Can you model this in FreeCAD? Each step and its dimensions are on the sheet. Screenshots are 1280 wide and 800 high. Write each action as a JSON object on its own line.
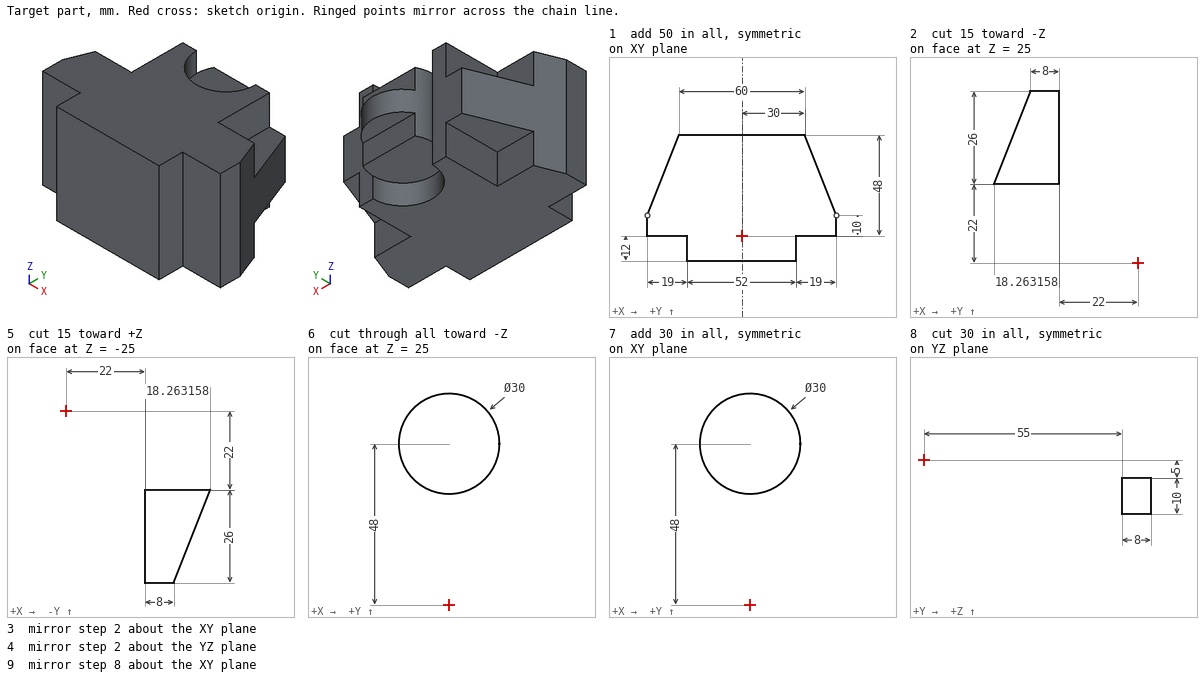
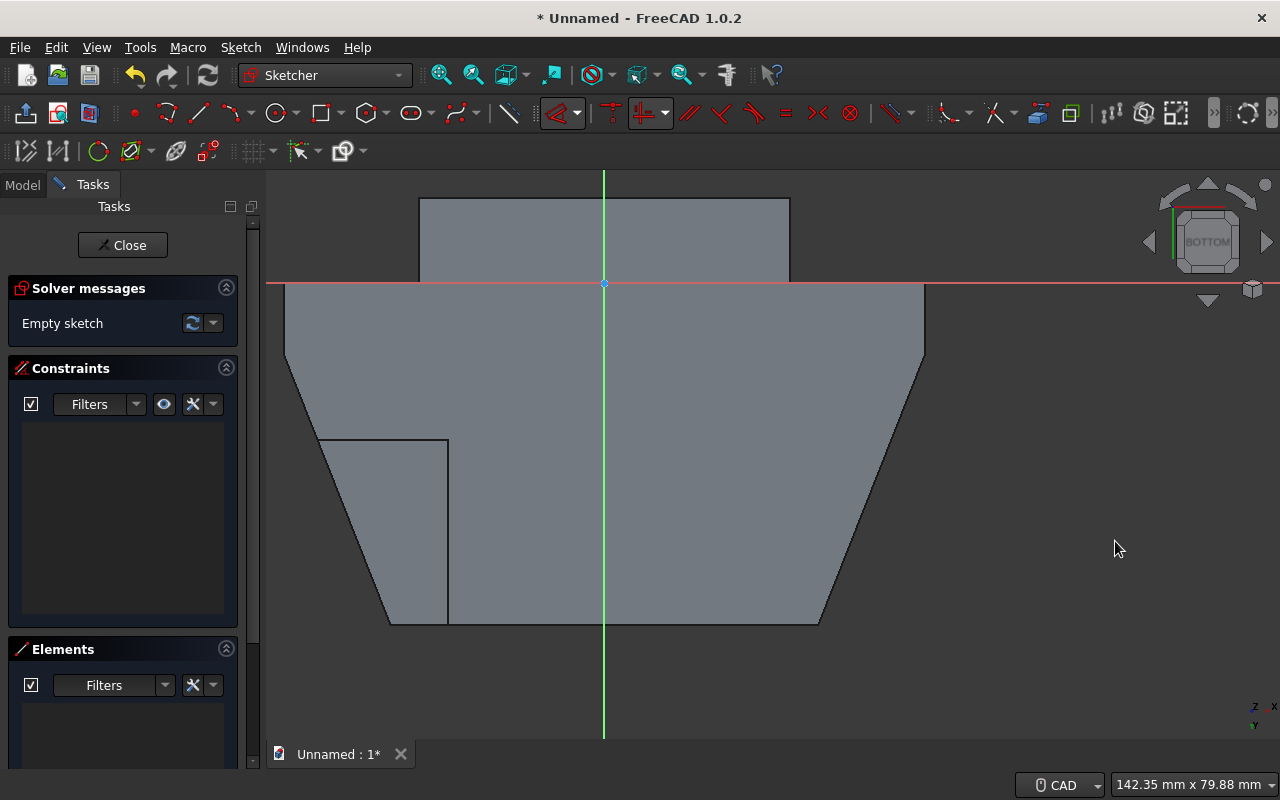
{"action": "left_click", "coordinate": [168, 114]}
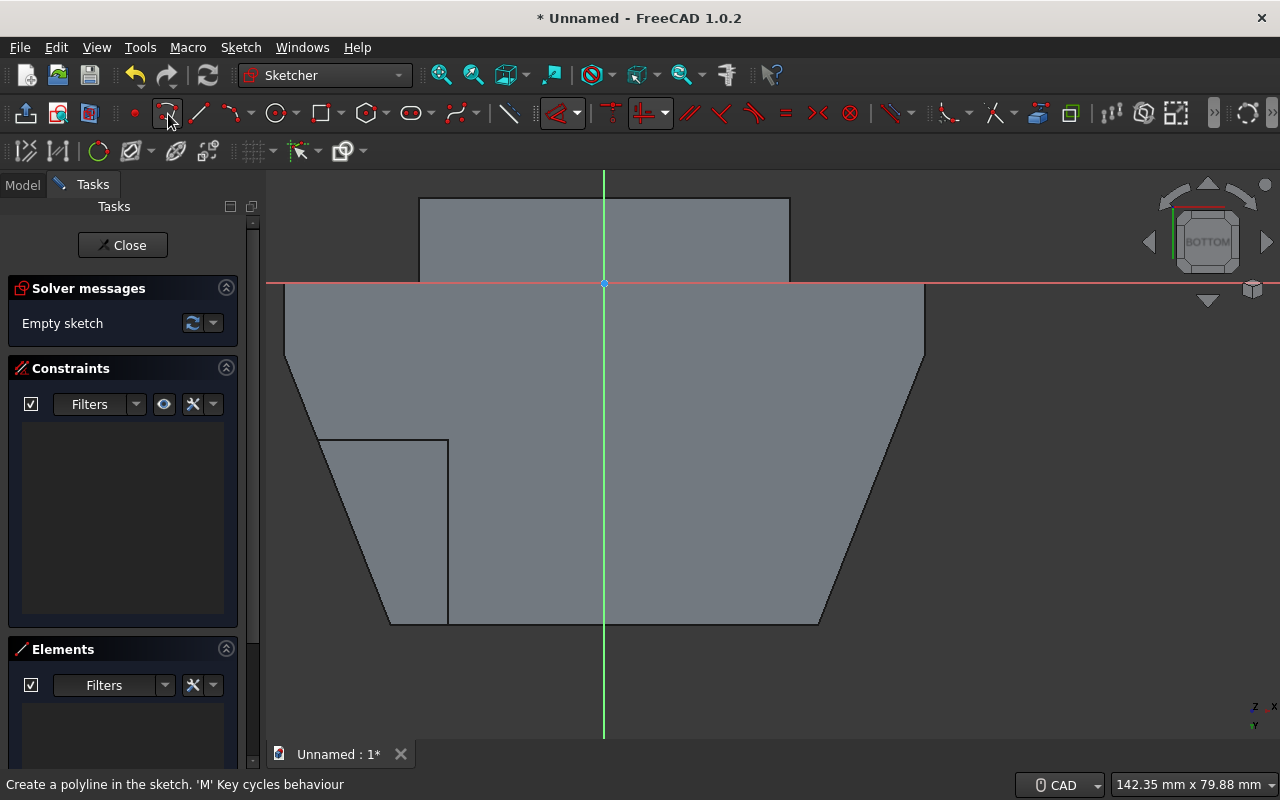
{"action": "left_click", "coordinate": [761, 440]}
{"action": "left_click", "coordinate": [761, 625]}
{"action": "left_click", "coordinate": [818, 625]}
{"action": "left_click", "coordinate": [891, 440]}
{"action": "left_click", "coordinate": [761, 441]}
{"action": "key", "text": "Escape"}
{"action": "key", "text": "Escape"}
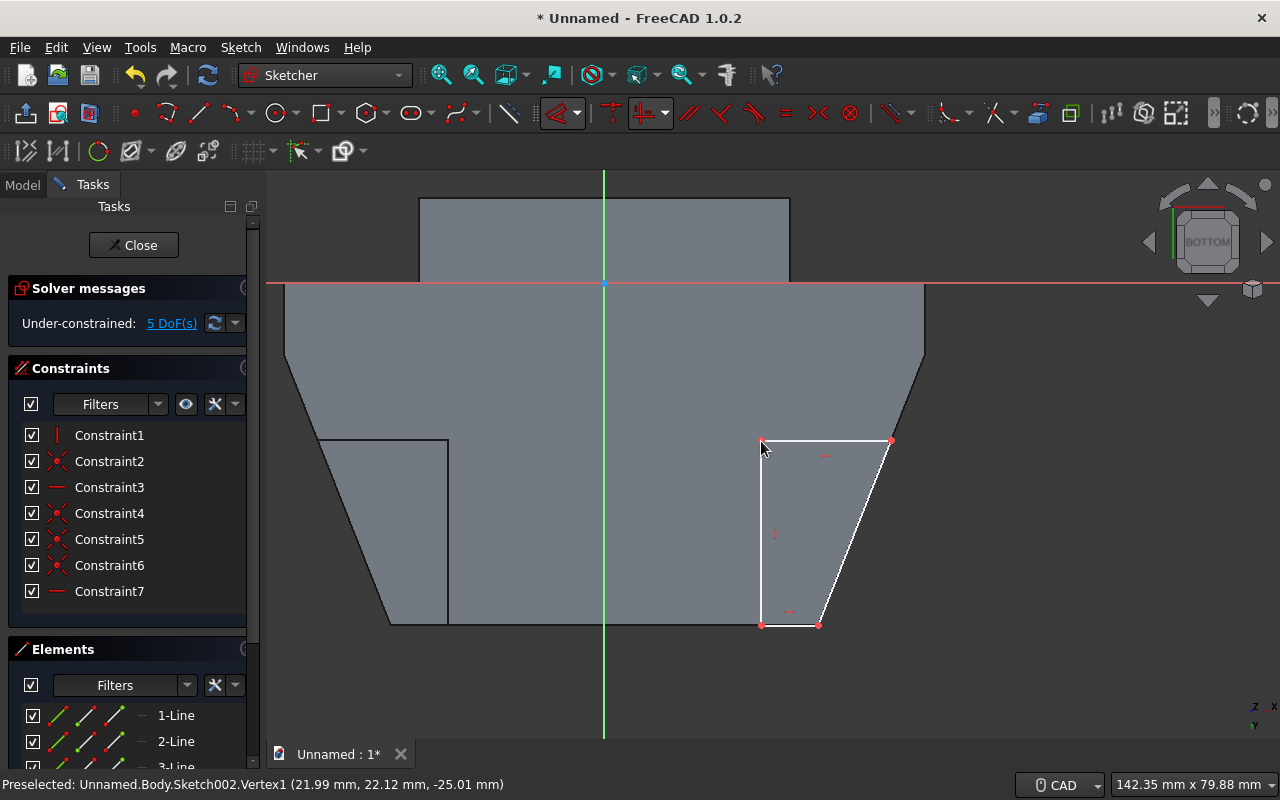
{"action": "left_click", "coordinate": [778, 626]}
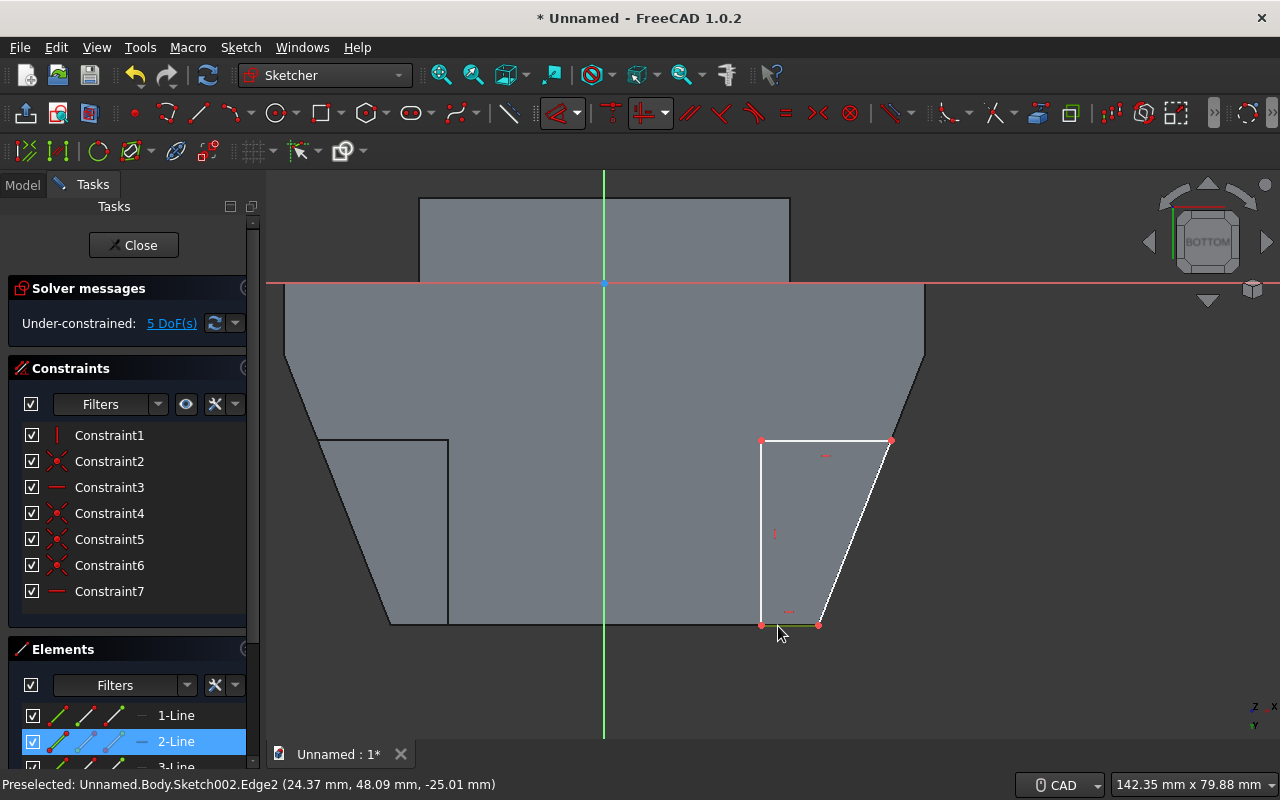
{"action": "left_click", "coordinate": [580, 114]}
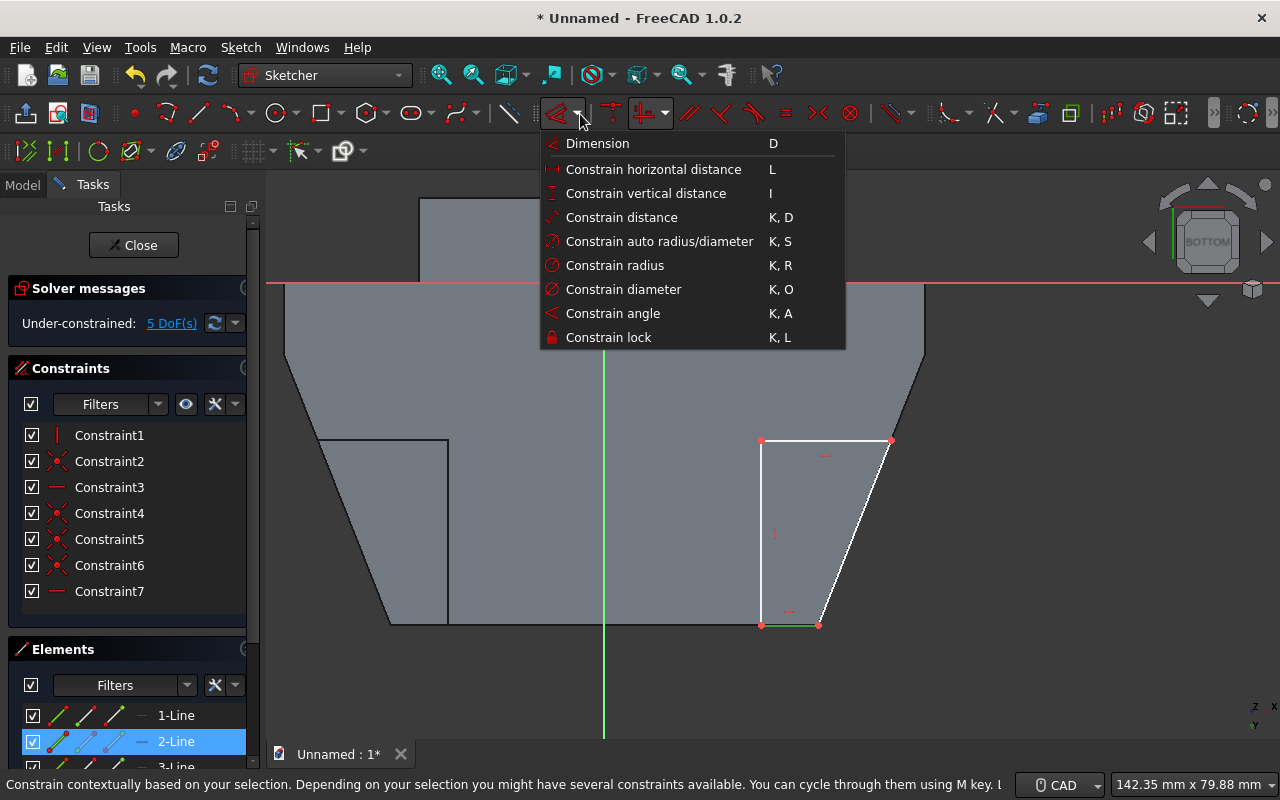
{"action": "left_click", "coordinate": [693, 169]}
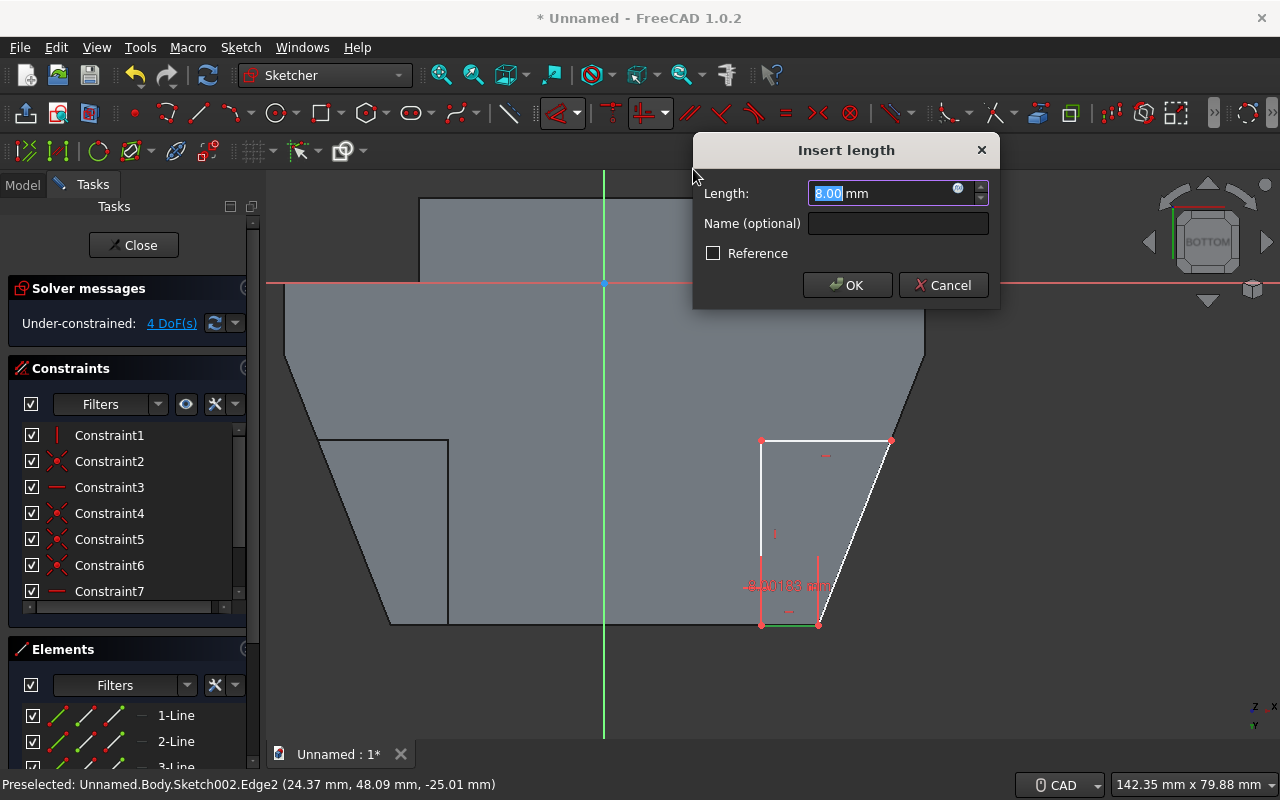
{"action": "type", "text": "8"}
{"action": "key", "text": "Return"}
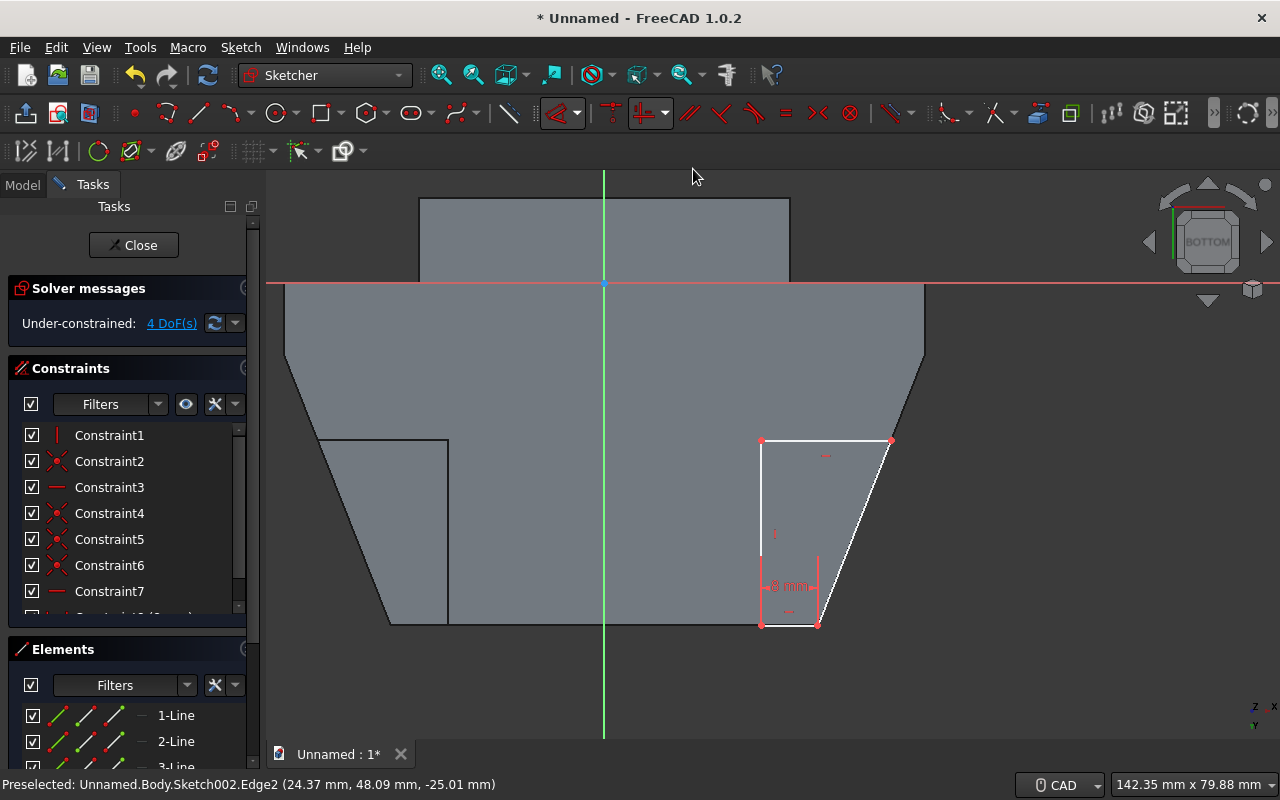
{"action": "left_click", "coordinate": [761, 497]}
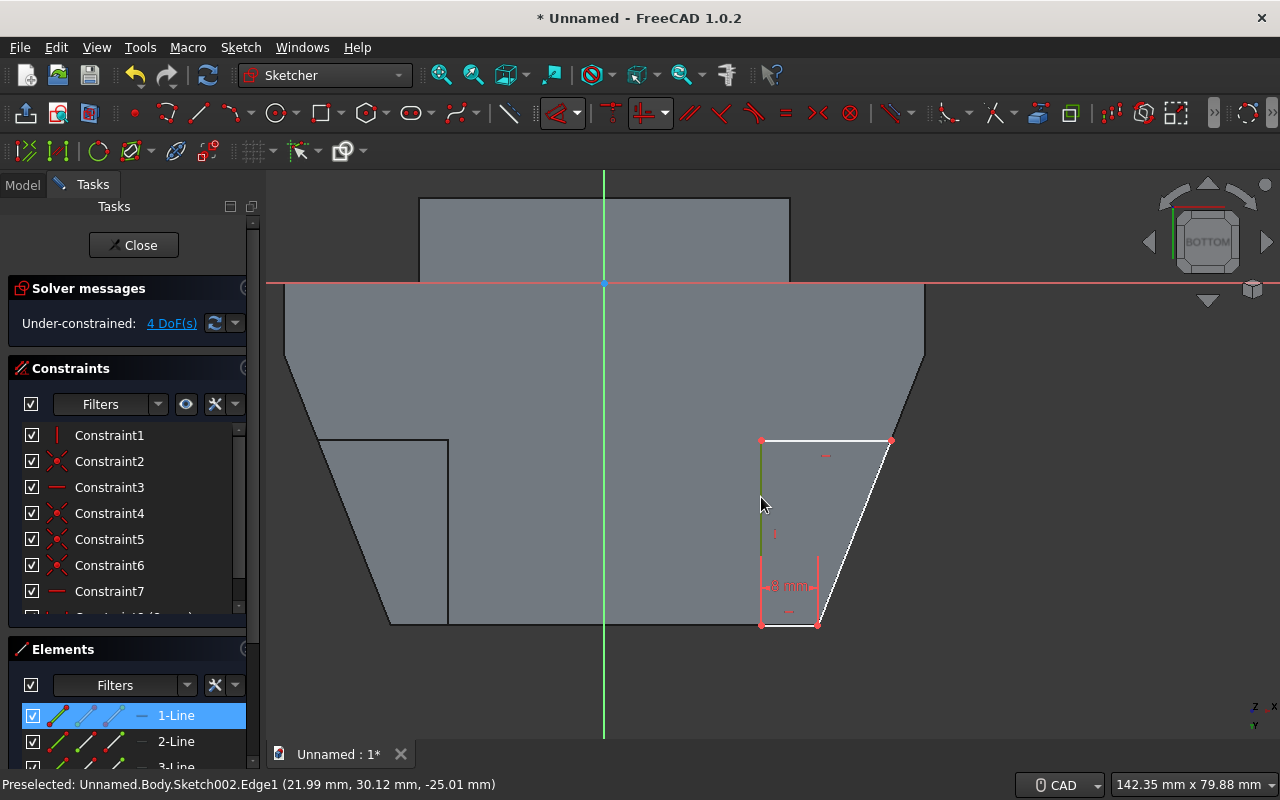
{"action": "left_click", "coordinate": [580, 114]}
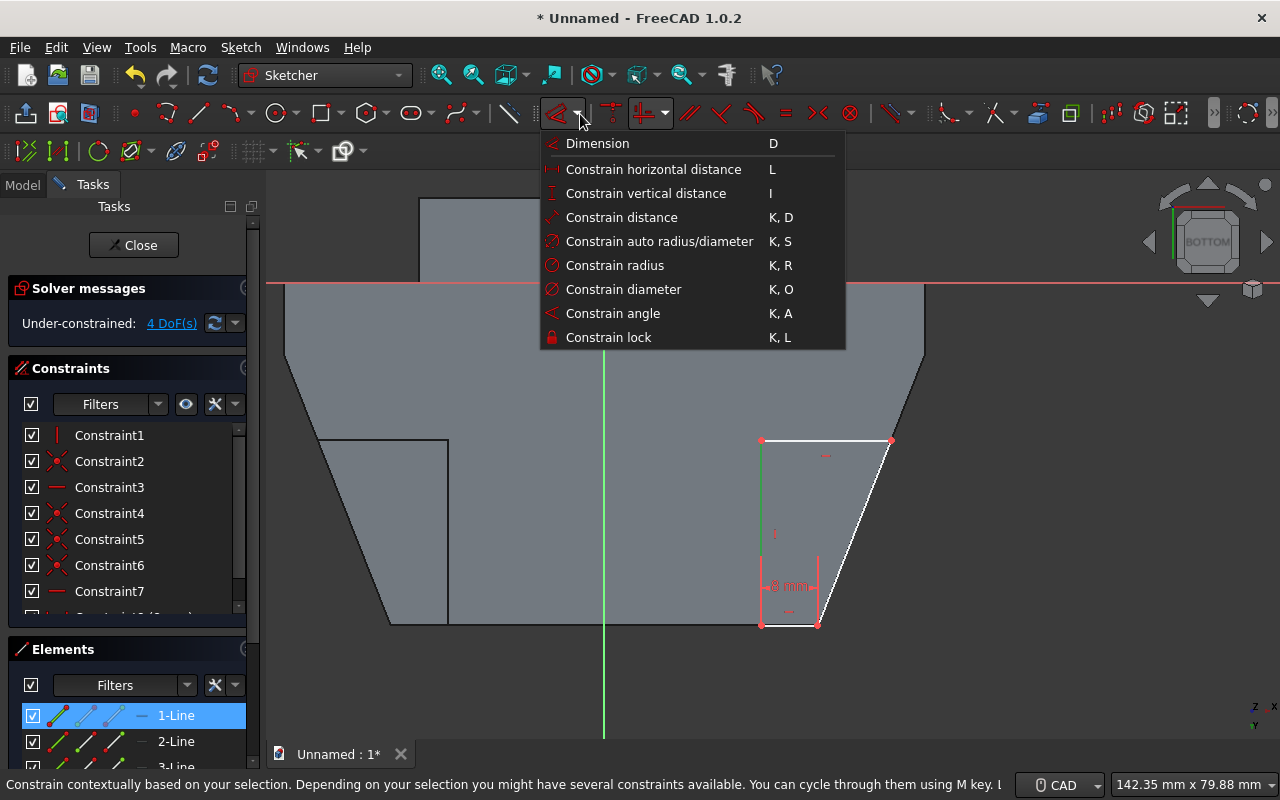
{"action": "left_click", "coordinate": [693, 193]}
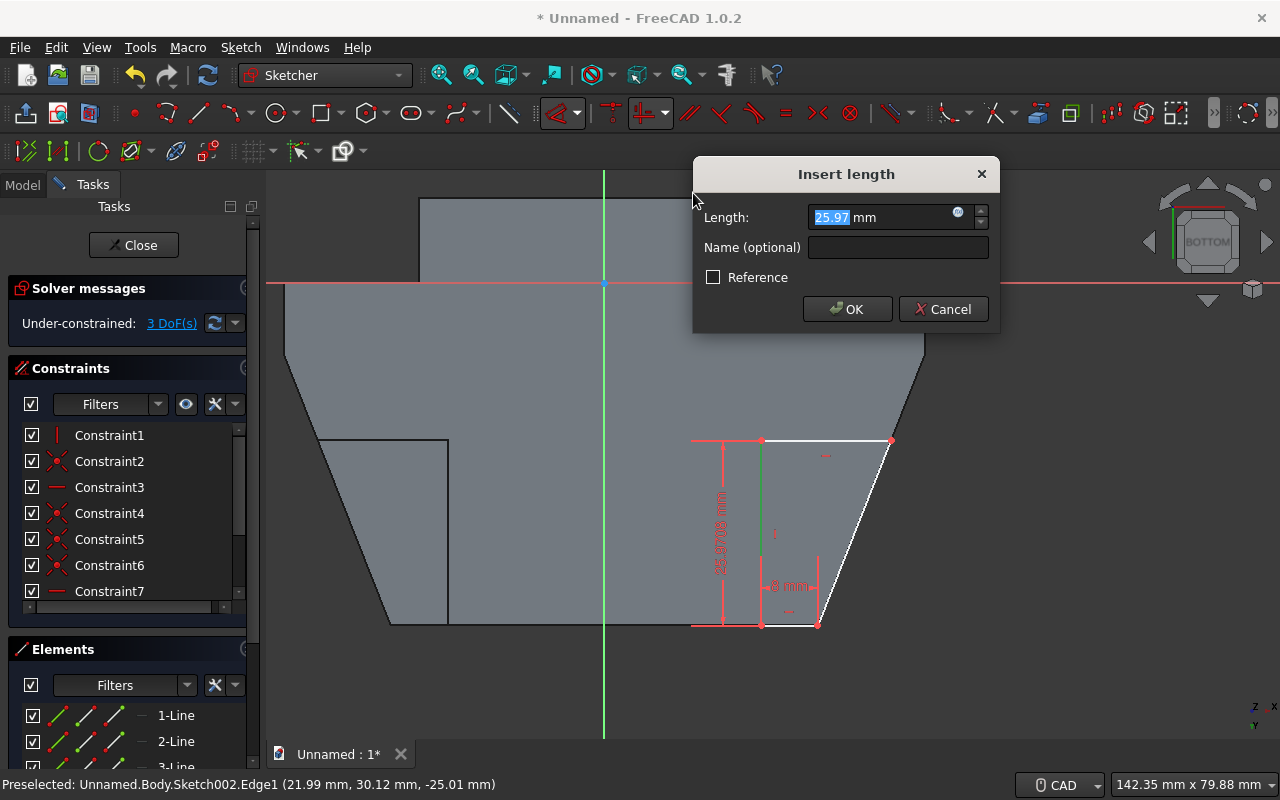
{"action": "type", "text": "26"}
{"action": "key", "text": "Return"}